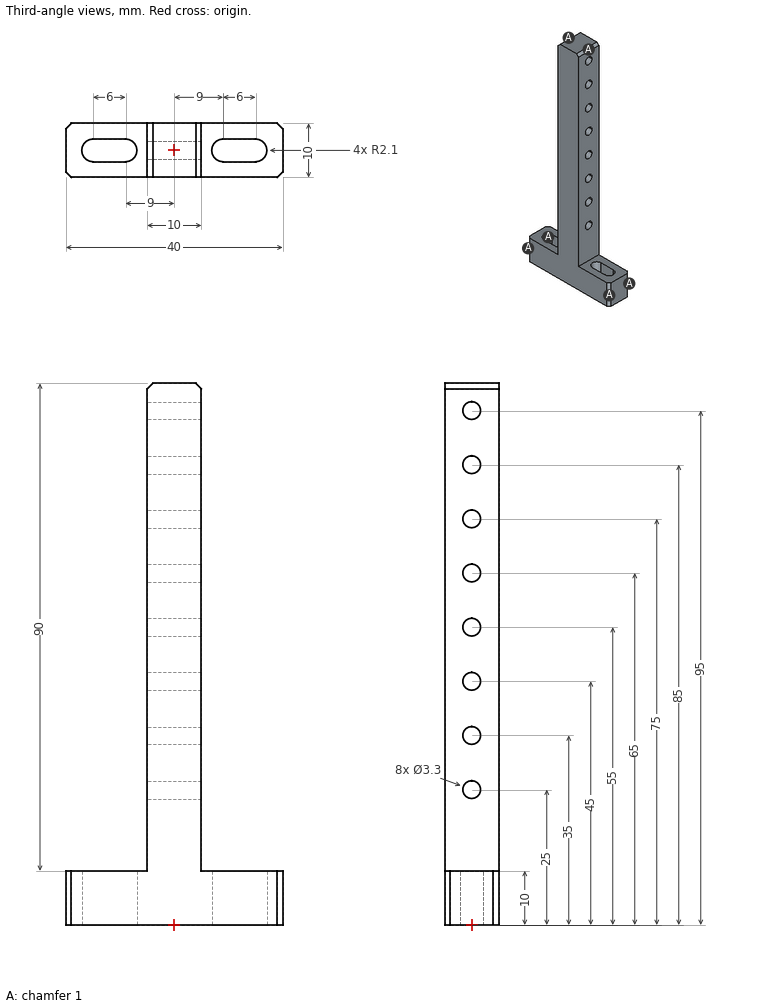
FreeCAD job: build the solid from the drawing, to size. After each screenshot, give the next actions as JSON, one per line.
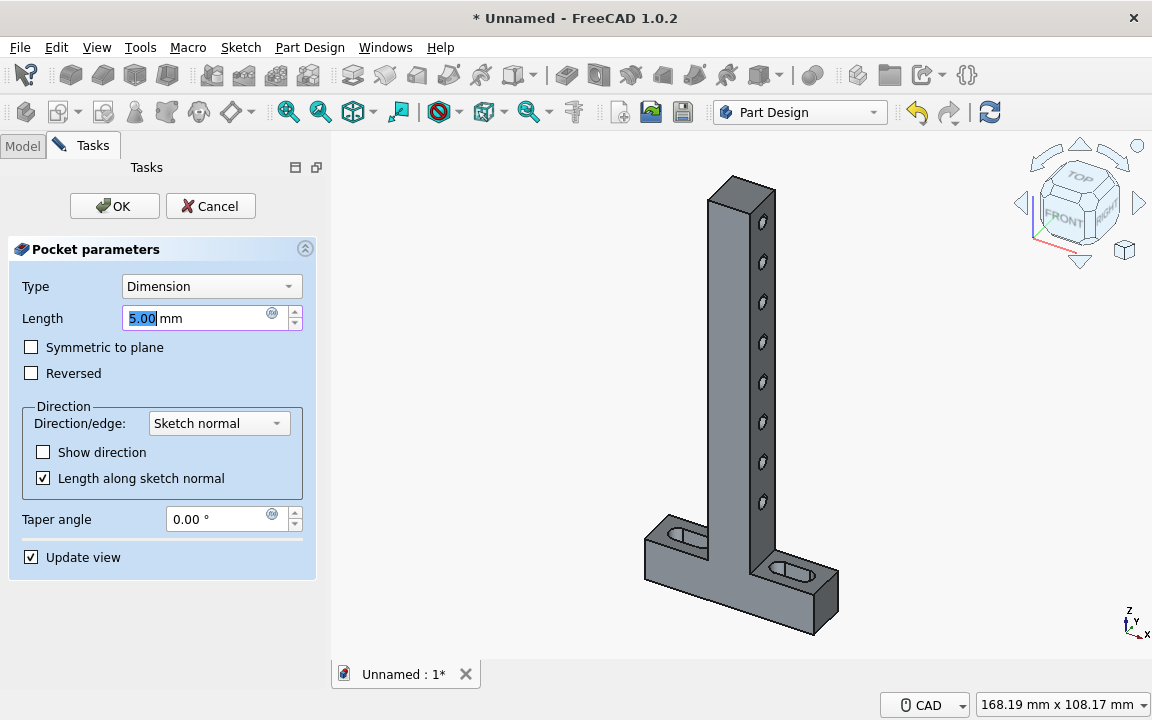
{"action": "left_click", "coordinate": [212, 286]}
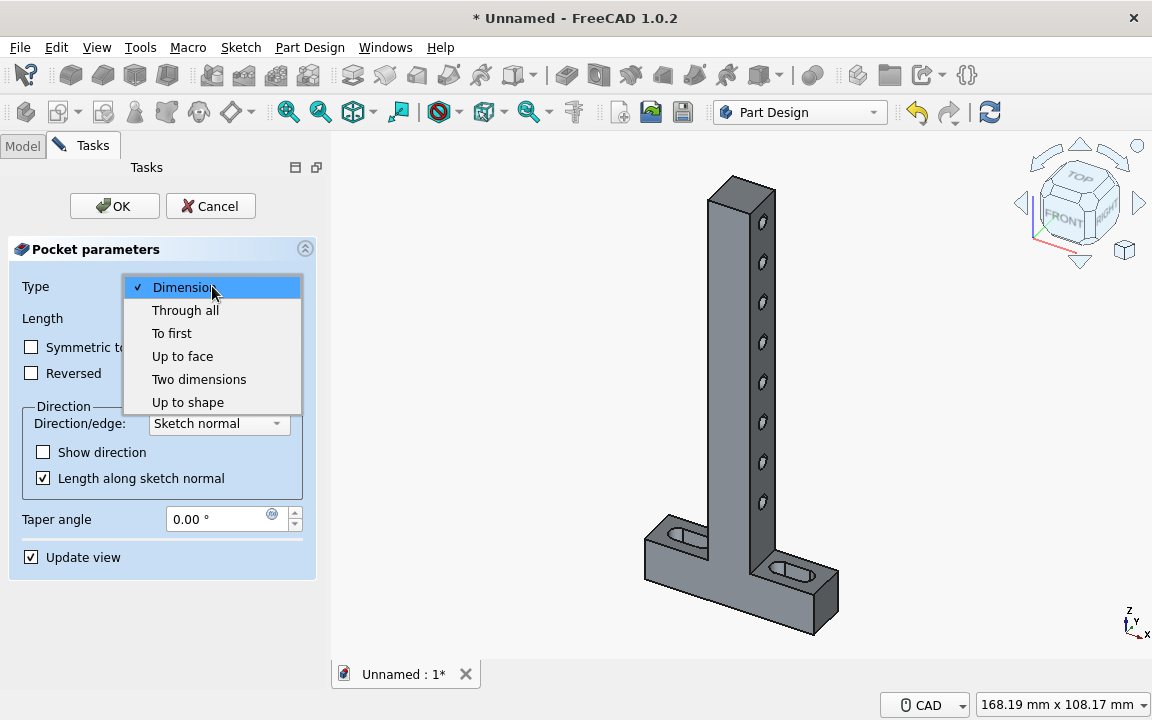
{"action": "left_click", "coordinate": [212, 310]}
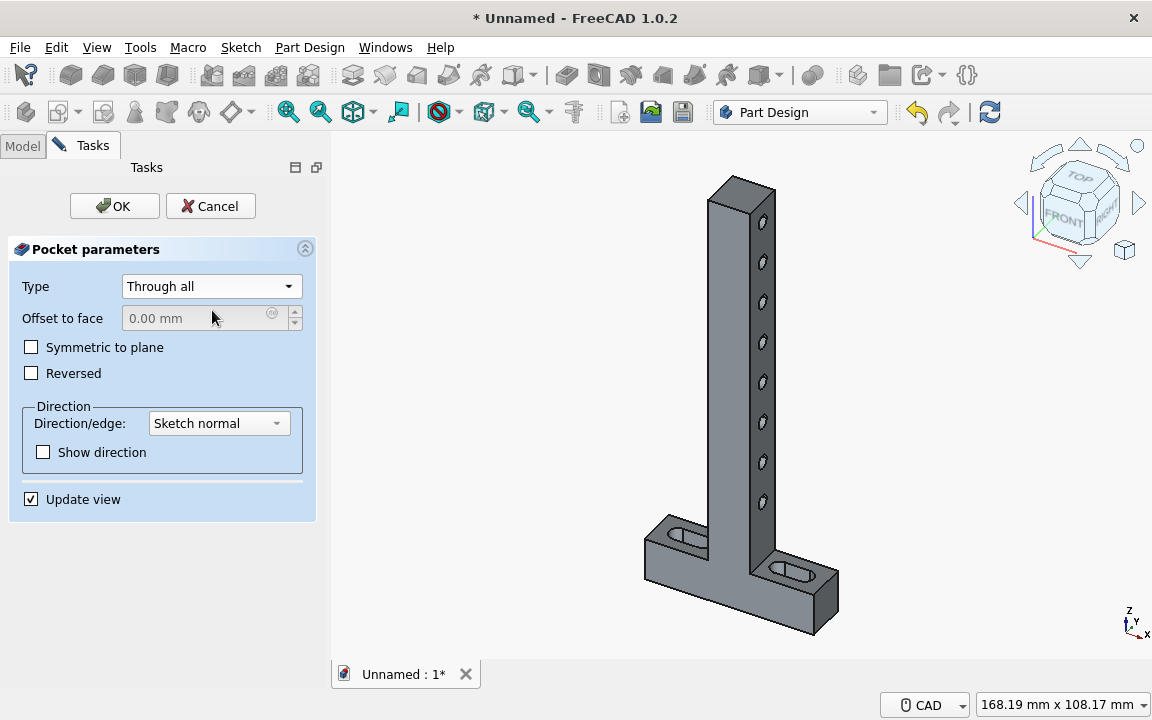
{"action": "left_click", "coordinate": [115, 206]}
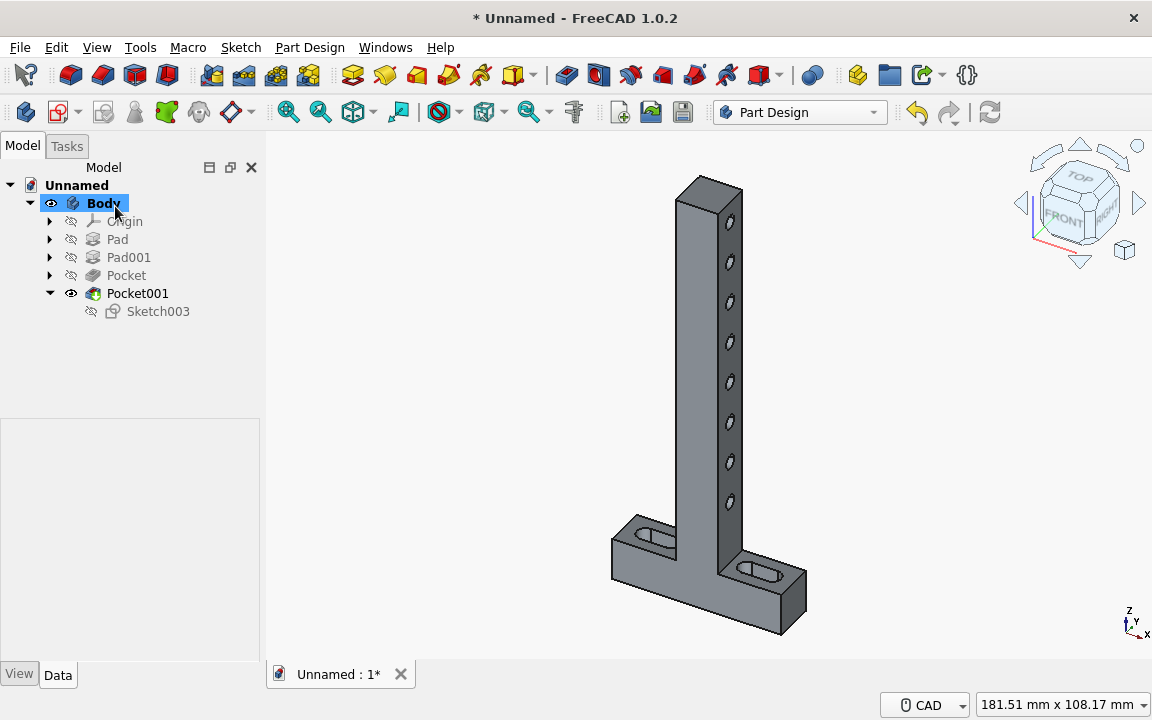
{"action": "left_click", "coordinate": [781, 614]}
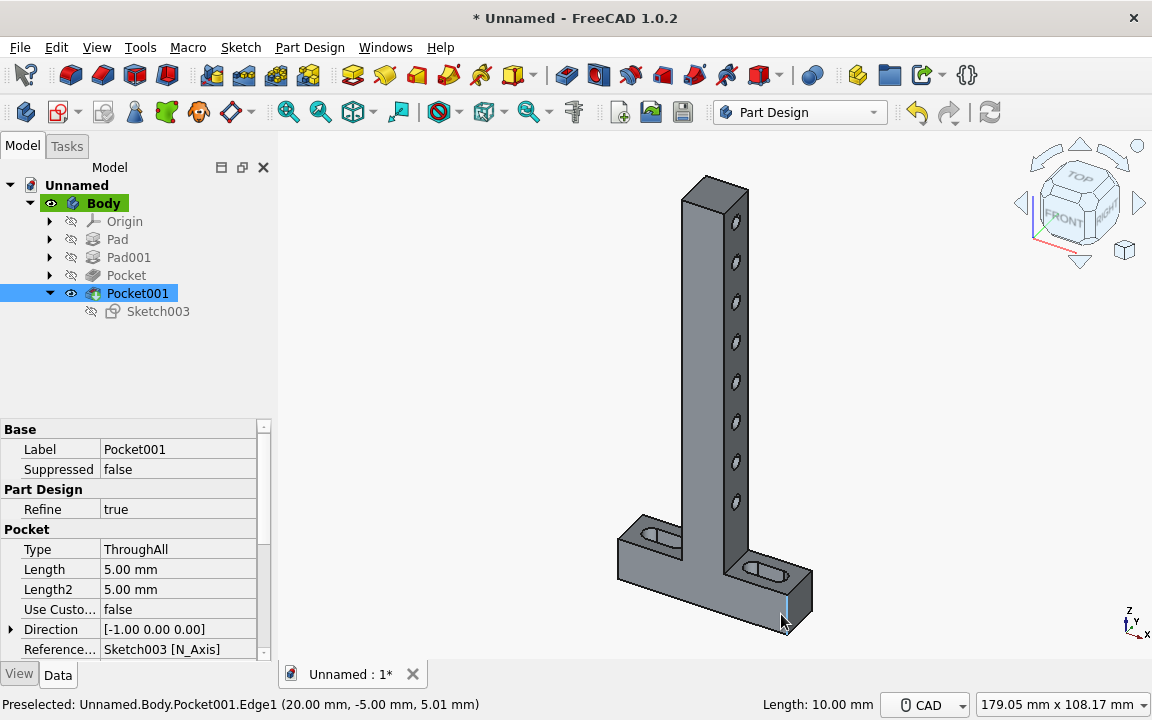
{"action": "left_click", "coordinate": [736, 201], "text": "ctrl"}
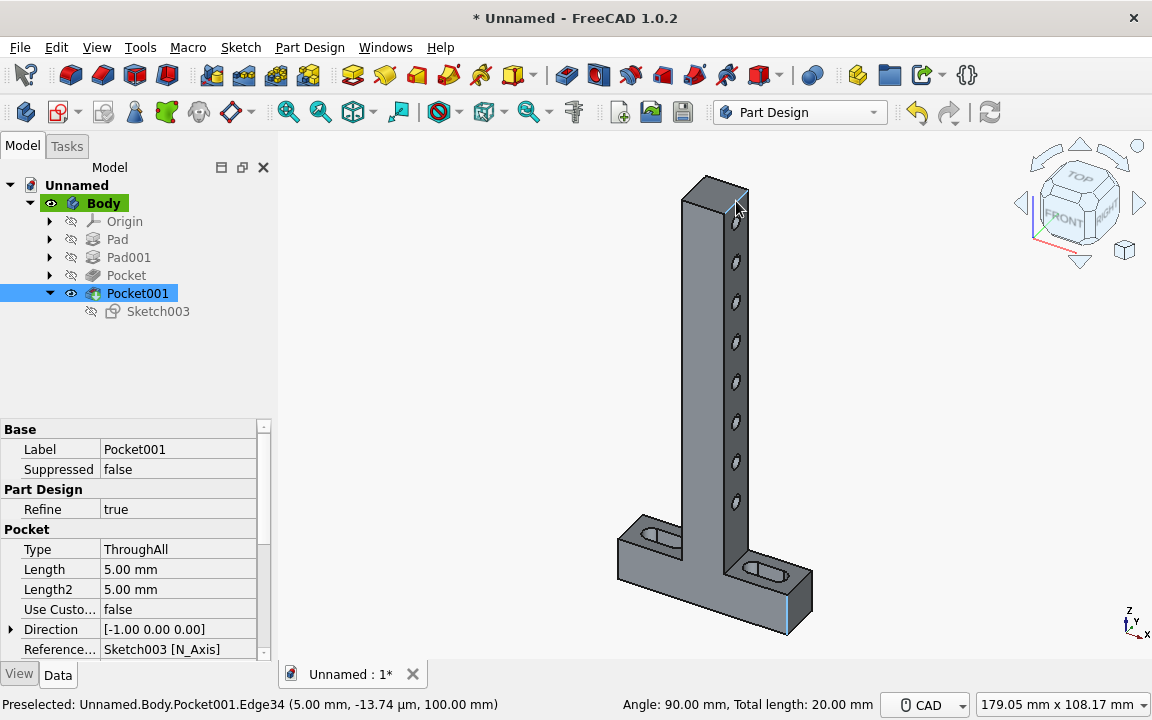
{"action": "key", "text": "0"}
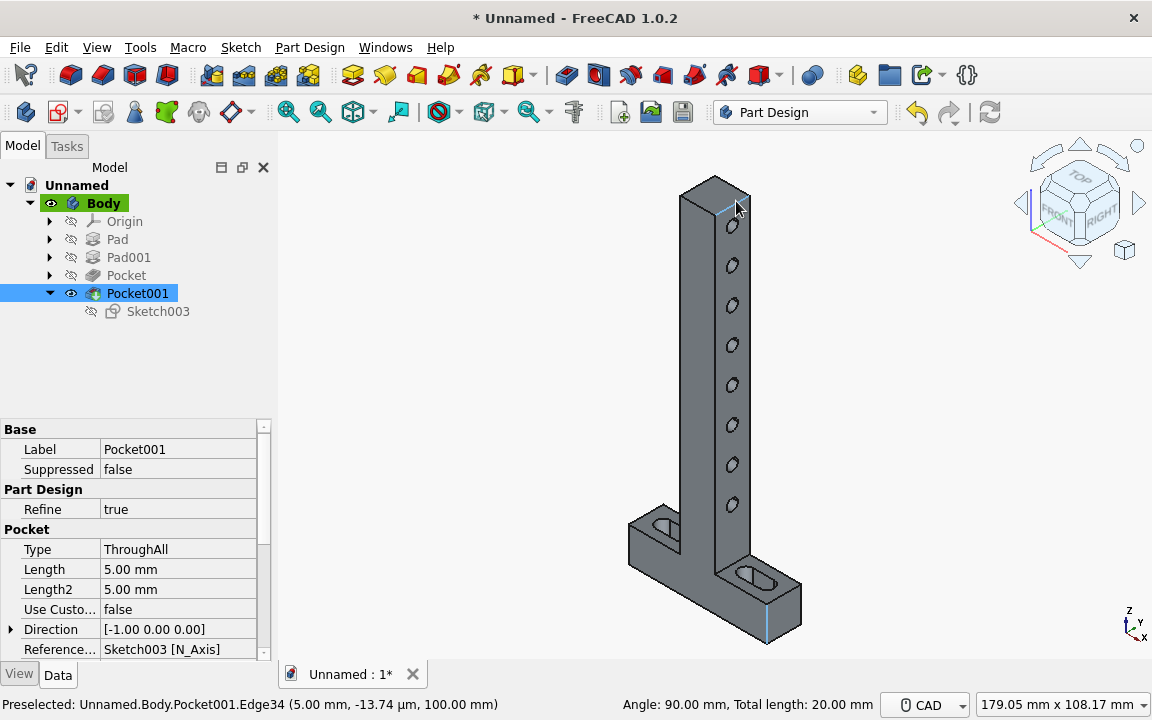
{"action": "key", "text": "2"}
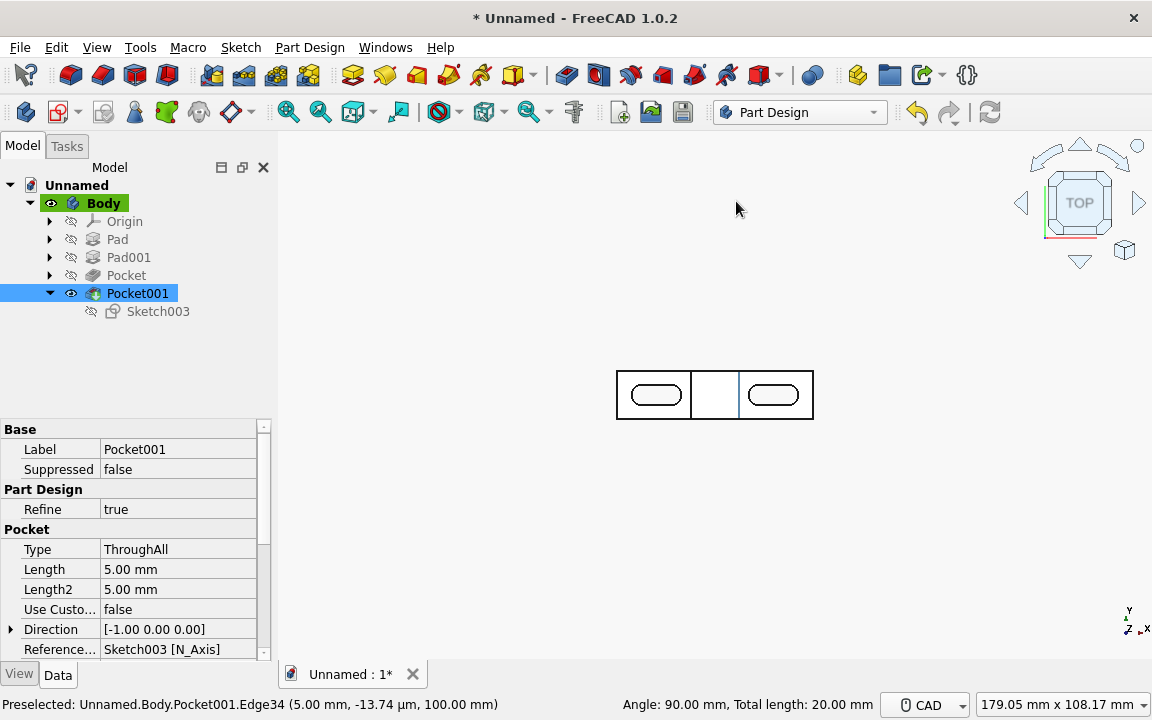
{"action": "left_click", "coordinate": [290, 112]}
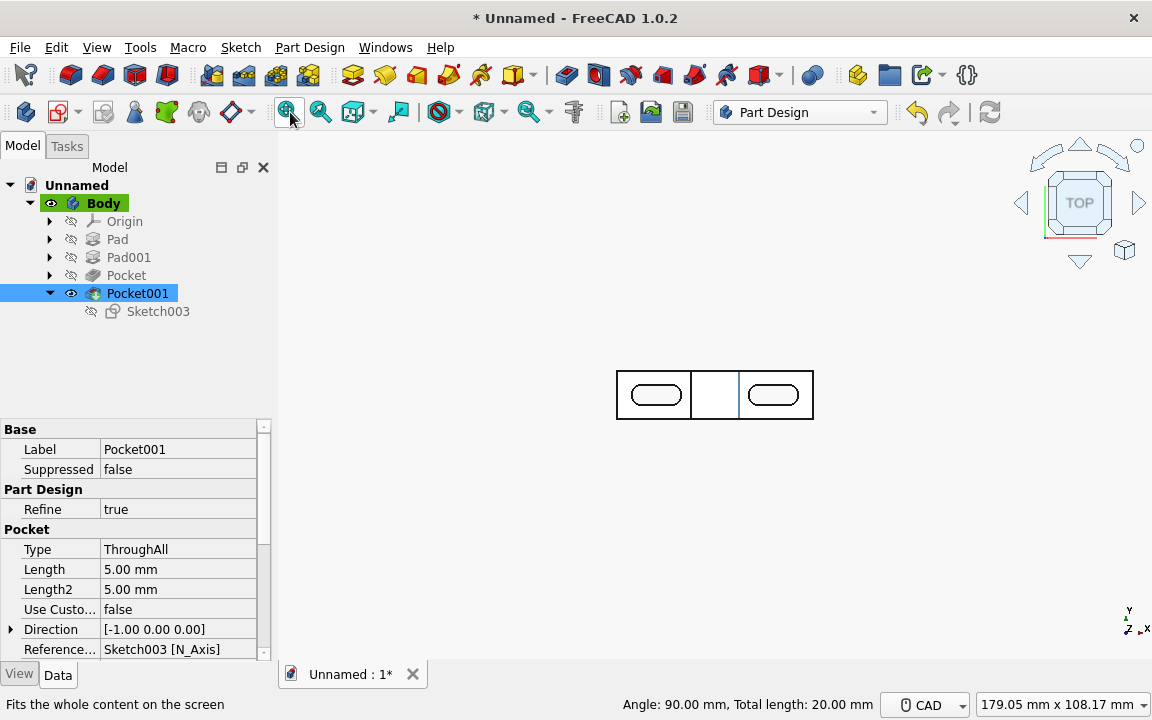
{"action": "left_click", "coordinate": [691, 394], "text": "ctrl"}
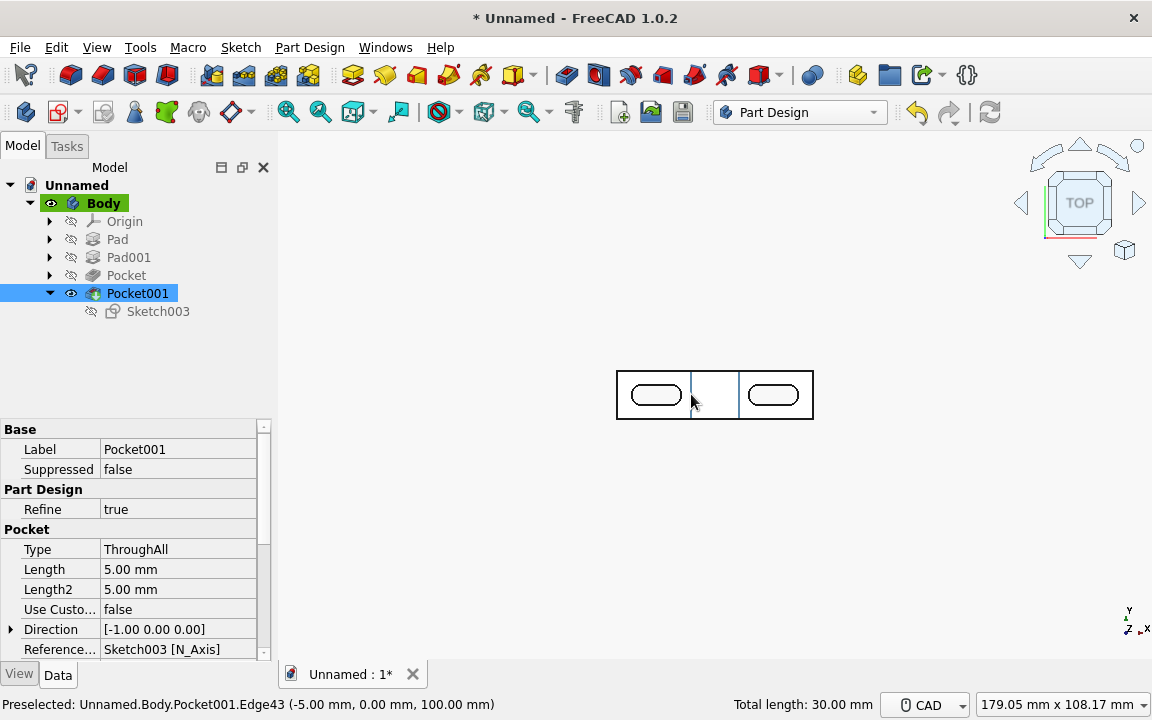
{"action": "key", "text": "1"}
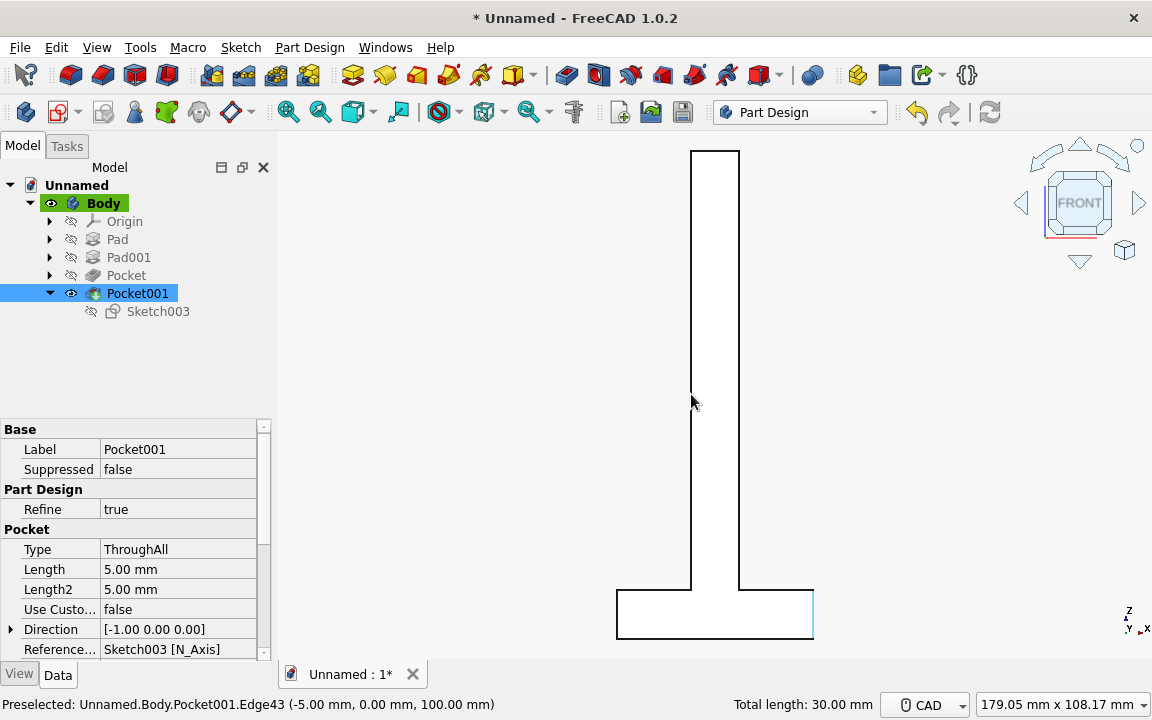
{"action": "left_click", "coordinate": [617, 614], "text": "ctrl"}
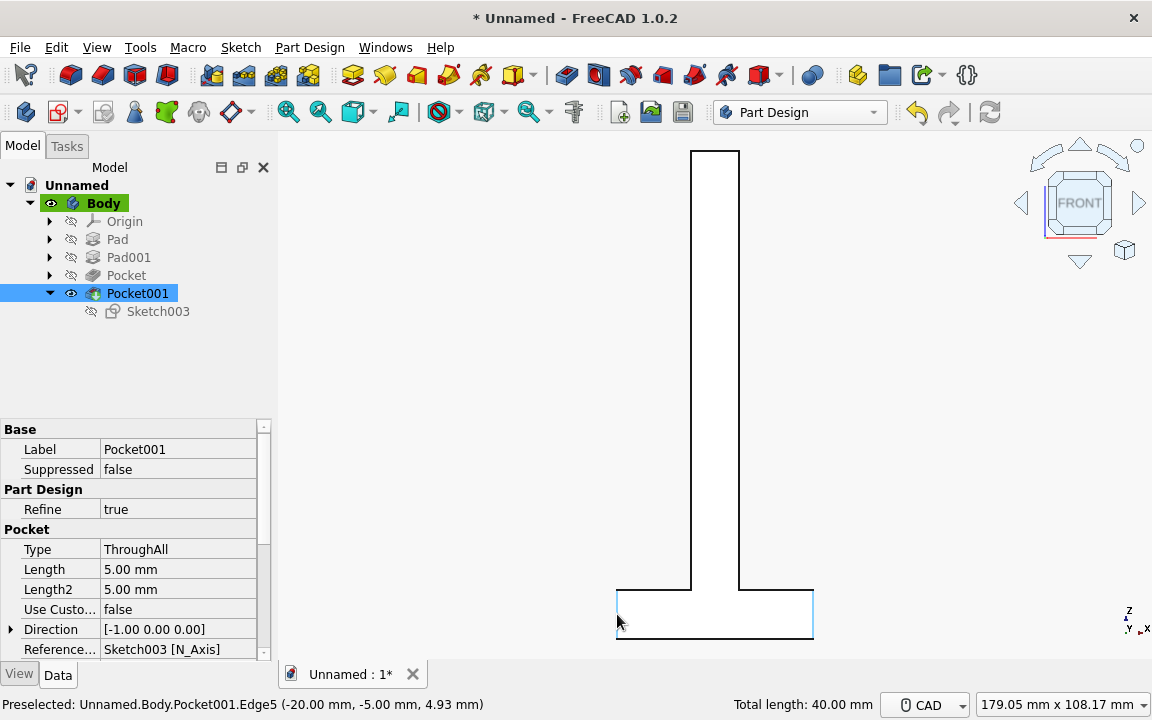
{"action": "key", "text": "3"}